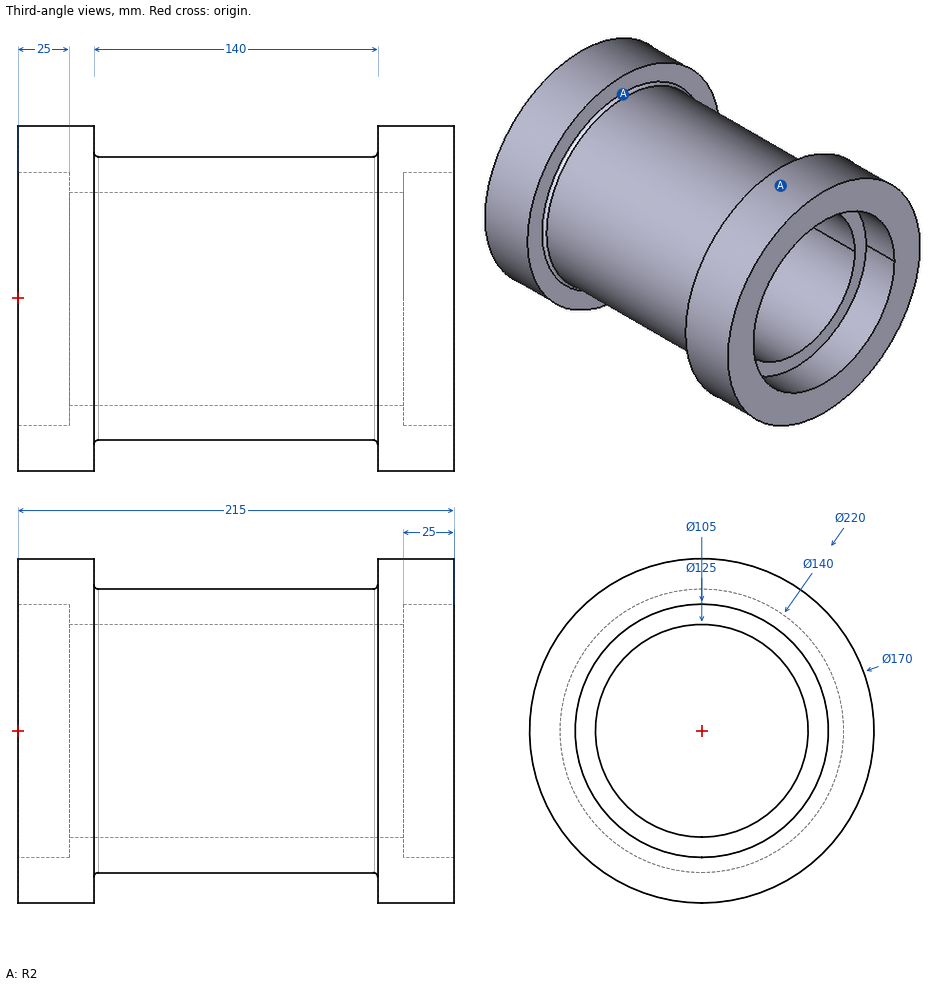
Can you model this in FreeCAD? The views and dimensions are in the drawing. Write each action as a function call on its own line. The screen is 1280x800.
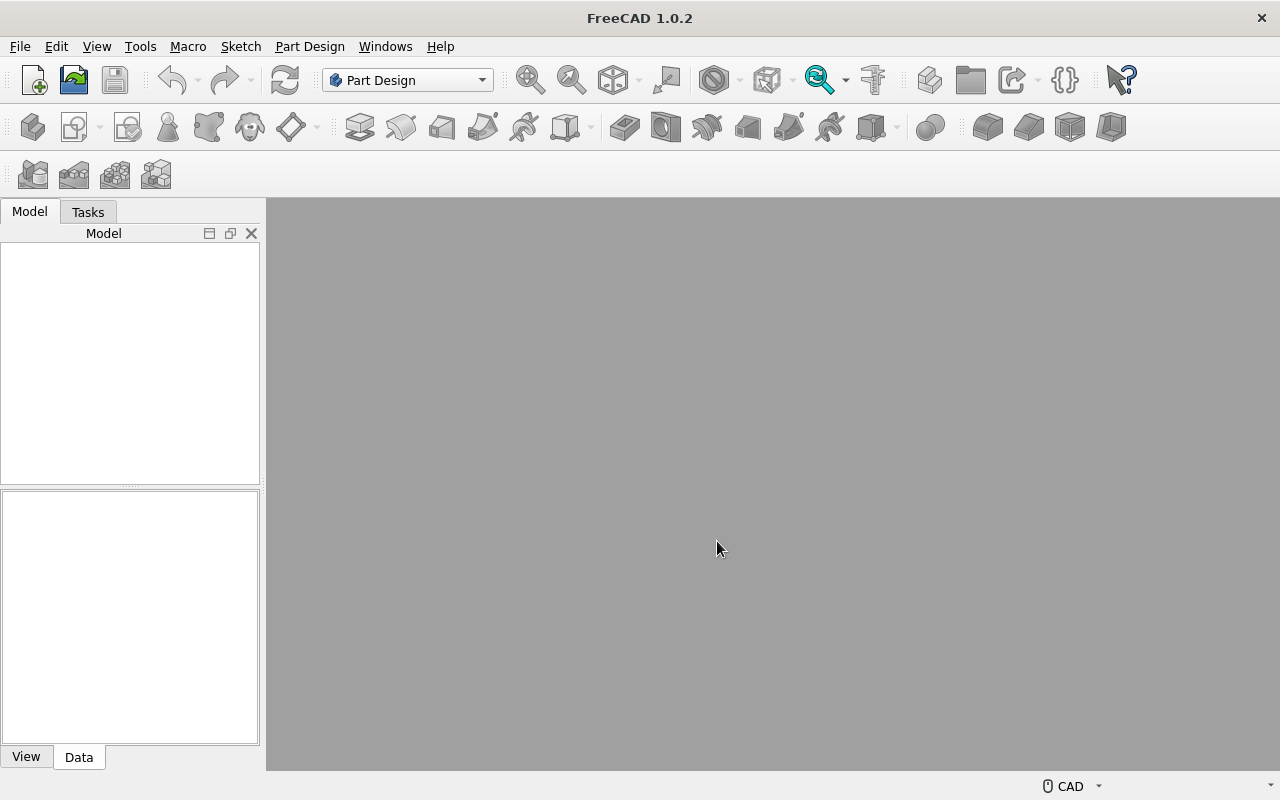
click(33, 80)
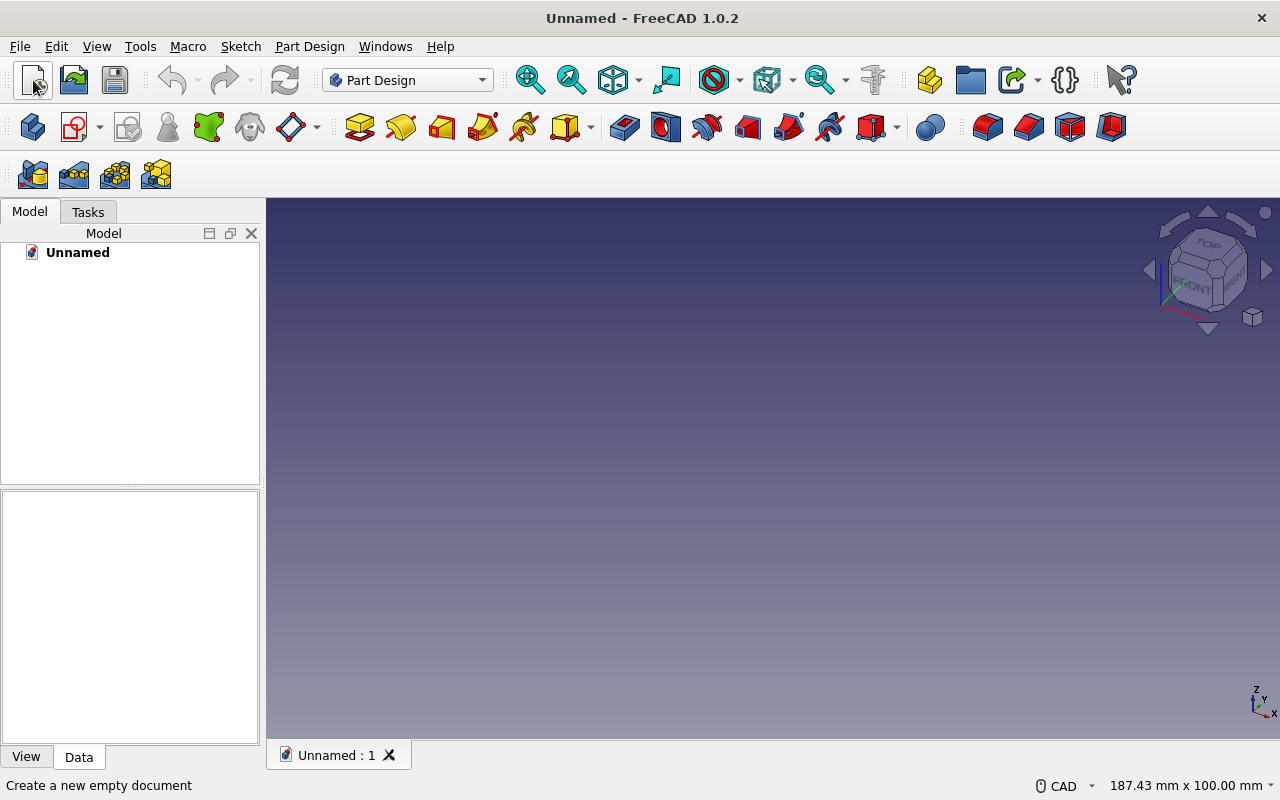
click(74, 128)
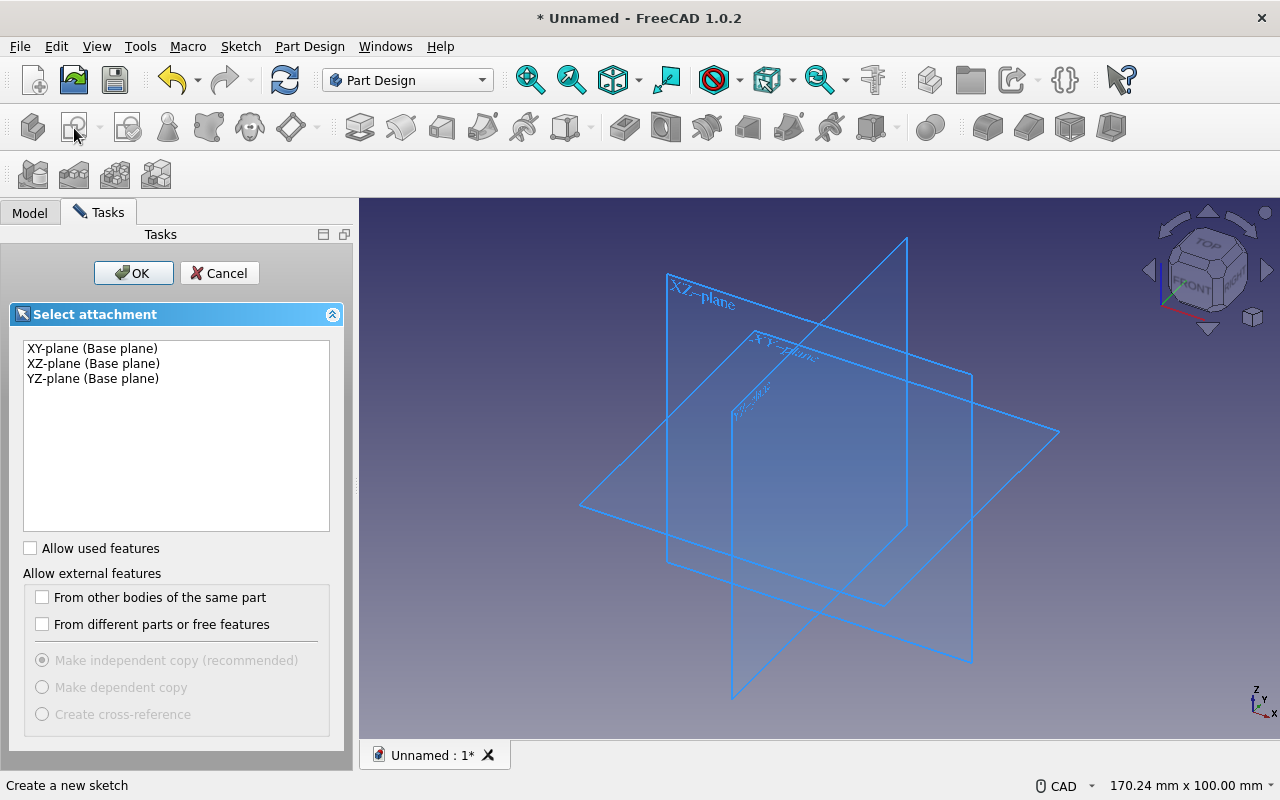
click(84, 378)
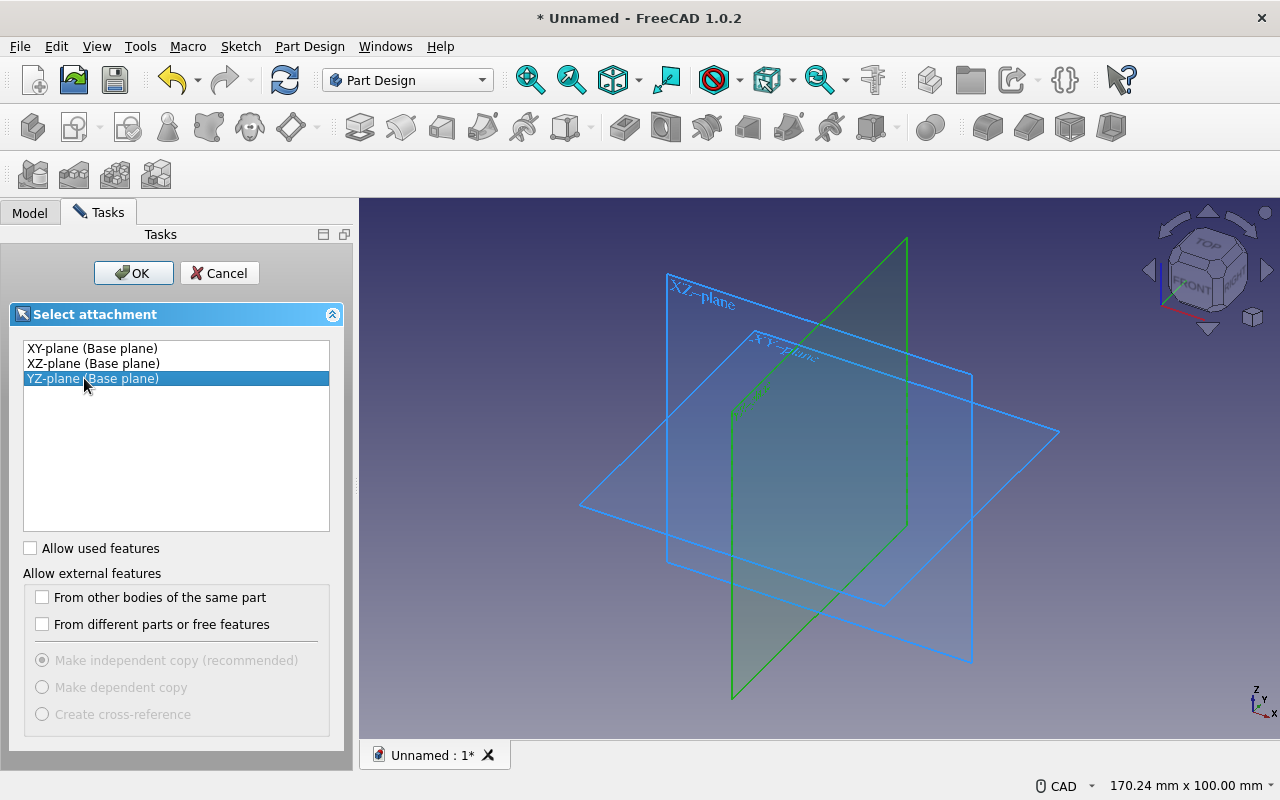
click(134, 273)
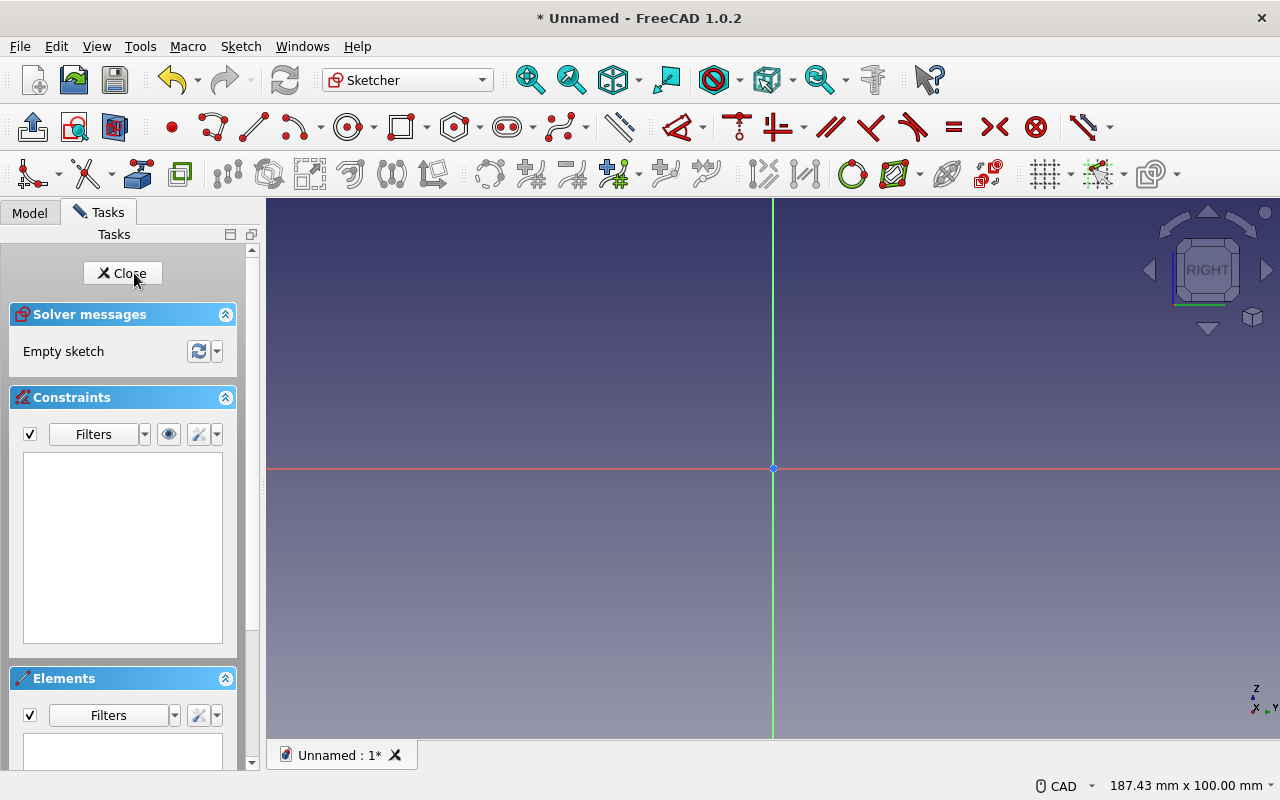
scroll(665, 469, down, 5)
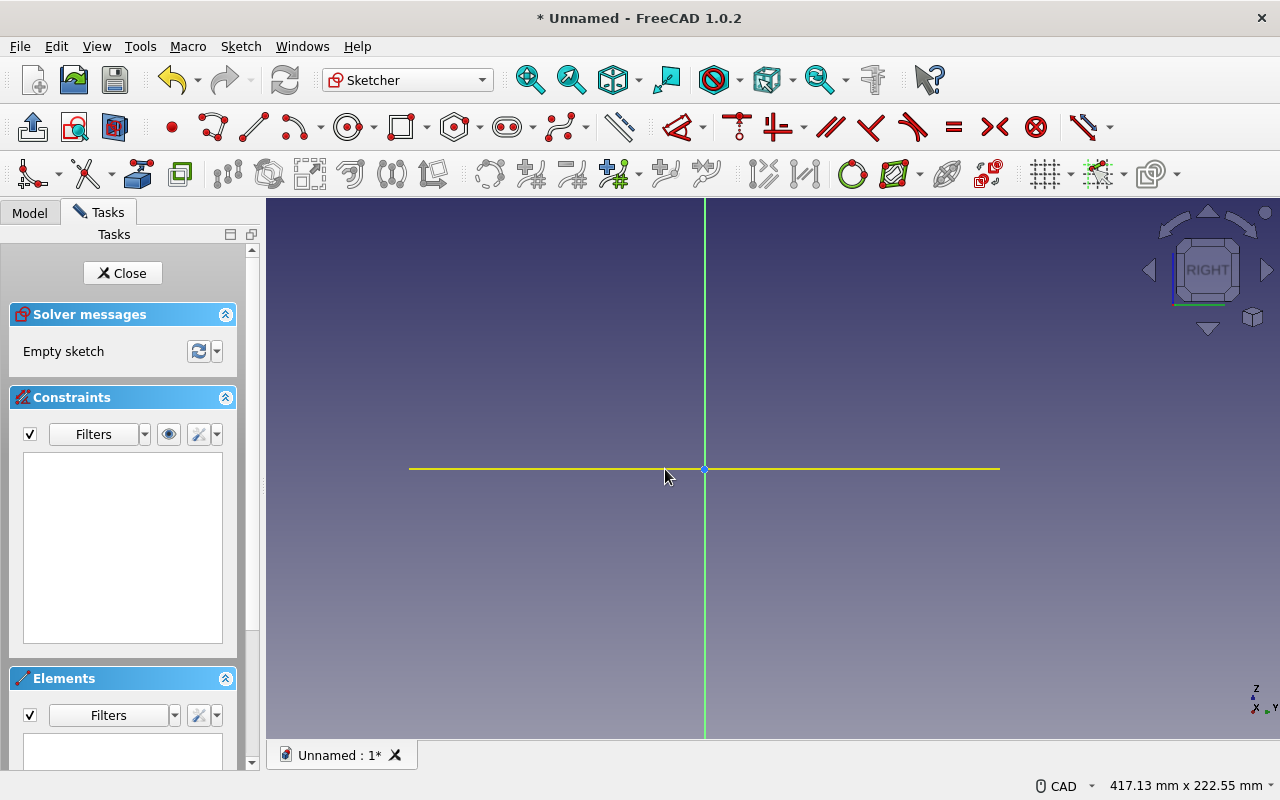
click(348, 128)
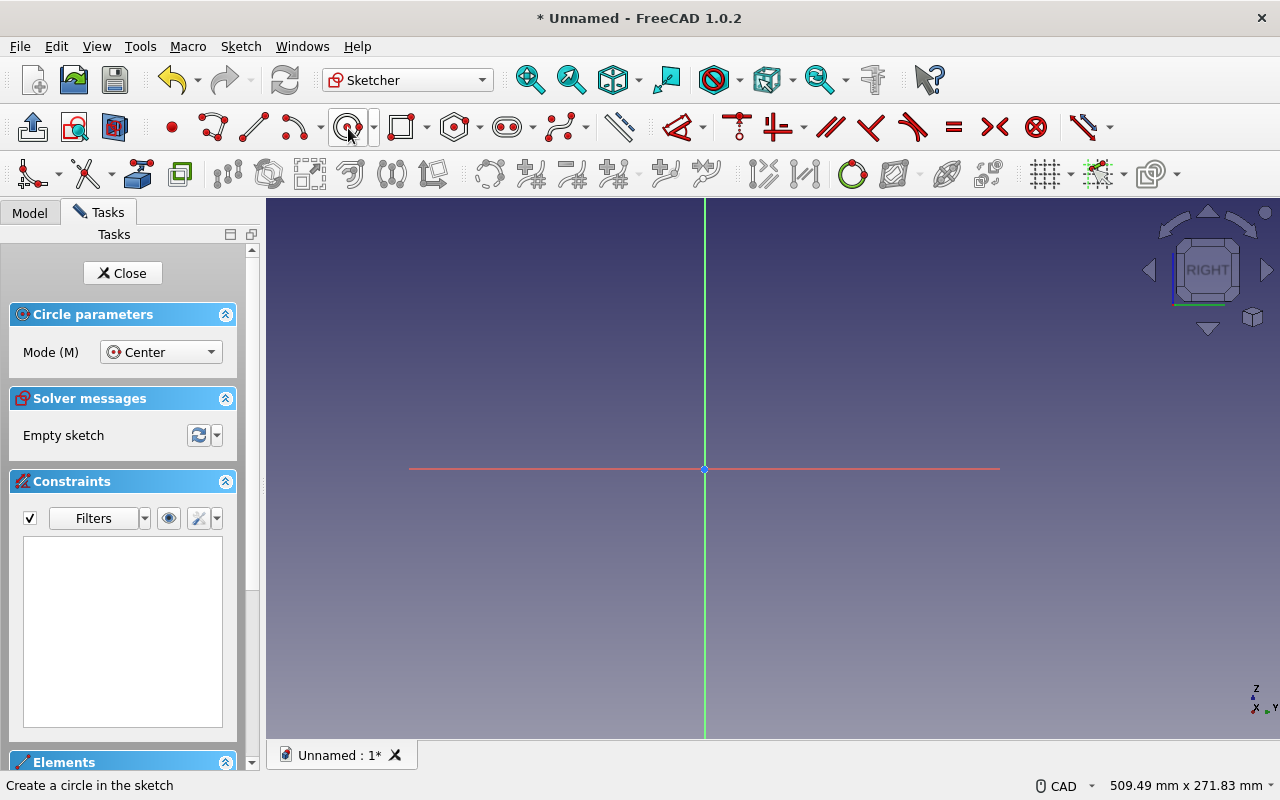
click(705, 469)
move(825, 350)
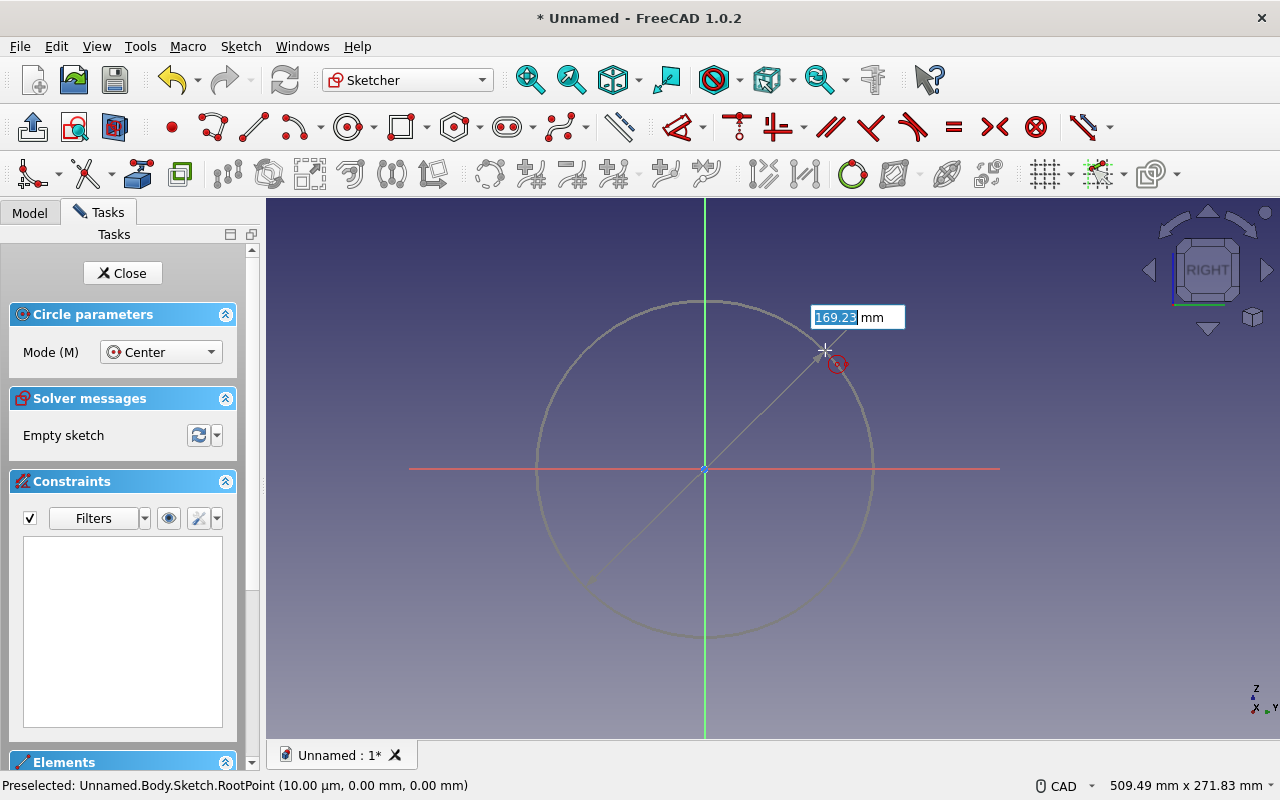
text(170)
key(Return)
key(Escape)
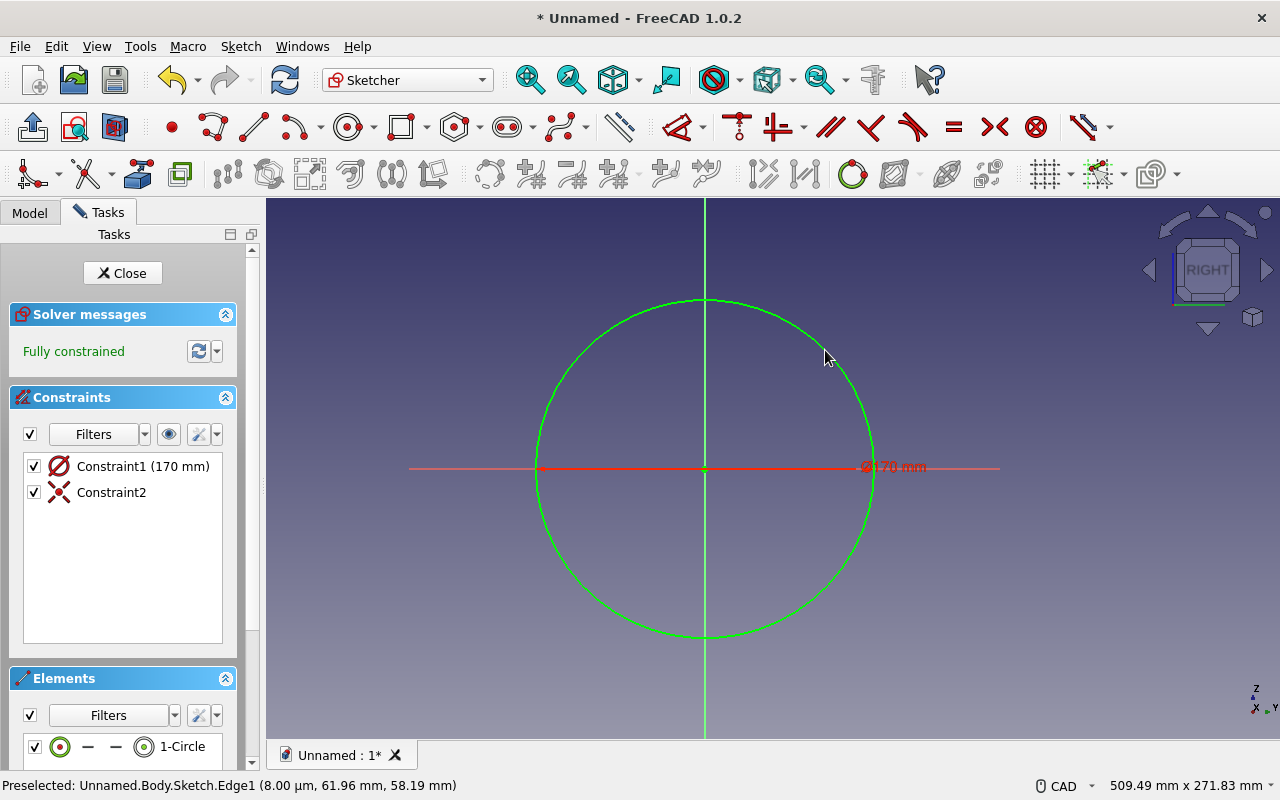
click(123, 273)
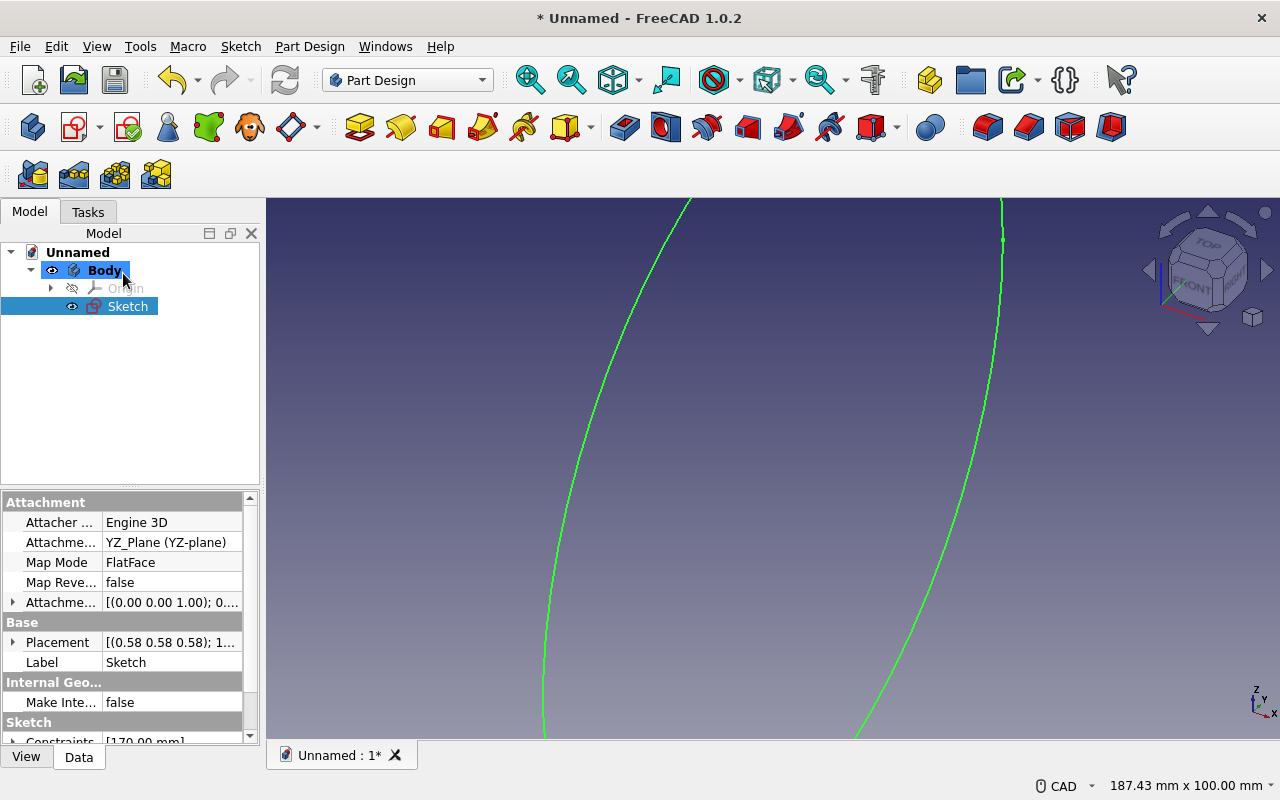
click(360, 128)